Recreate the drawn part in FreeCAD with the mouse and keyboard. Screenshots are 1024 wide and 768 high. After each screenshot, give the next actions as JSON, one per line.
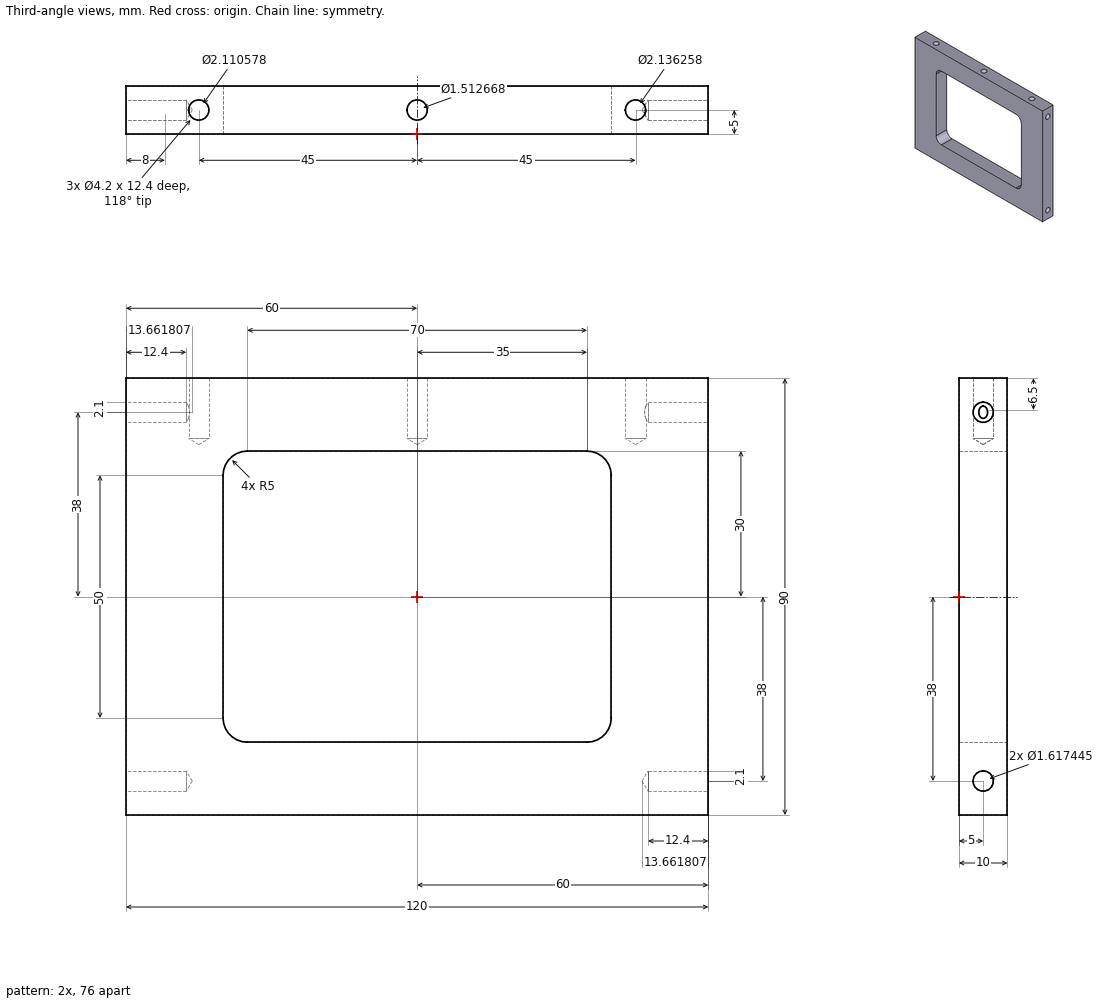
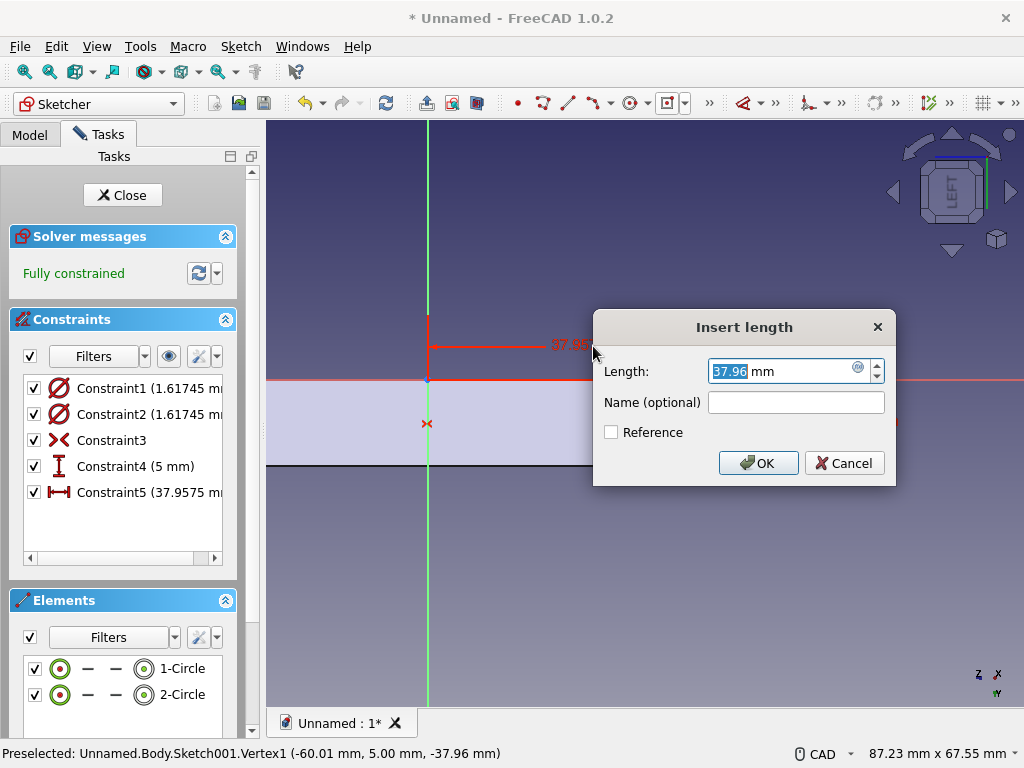
{"action": "type", "text": "38"}
{"action": "key", "text": "Return"}
{"action": "key", "text": "Escape"}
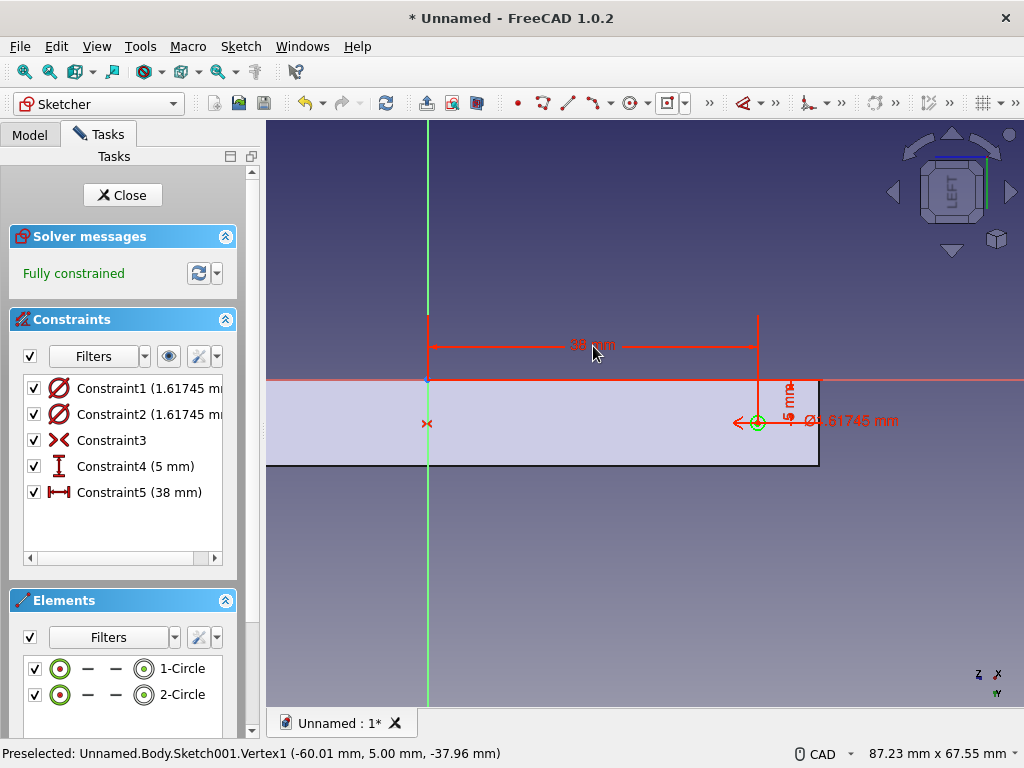
{"action": "left_click", "coordinate": [123, 195]}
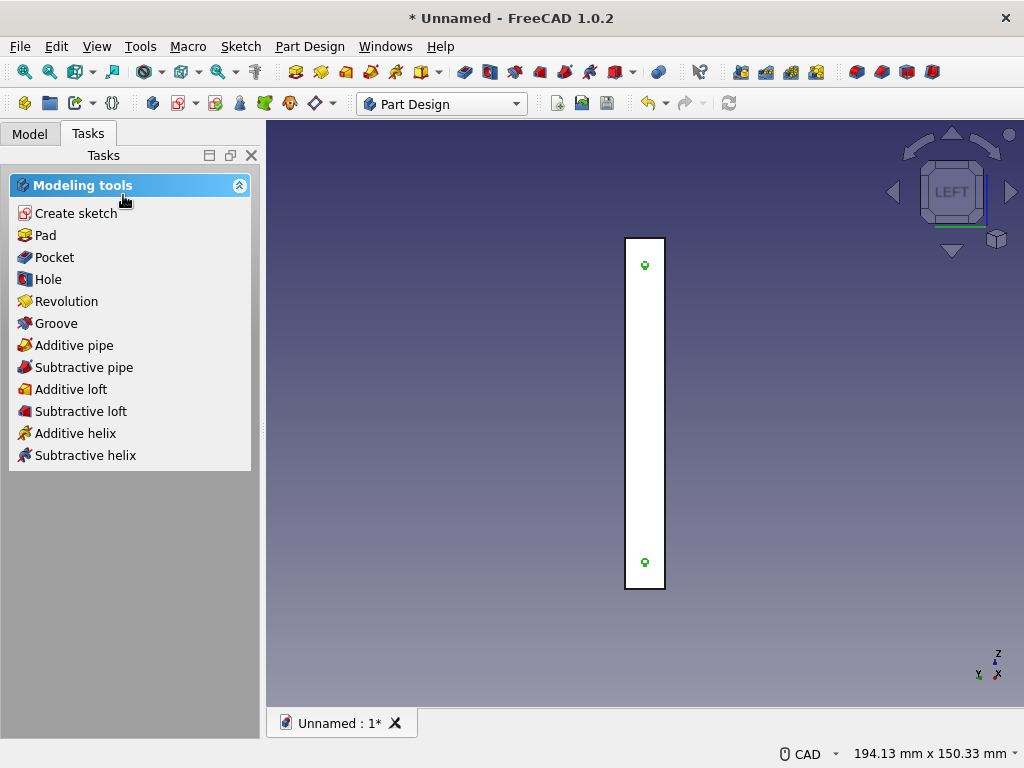
{"action": "left_click", "coordinate": [465, 72]}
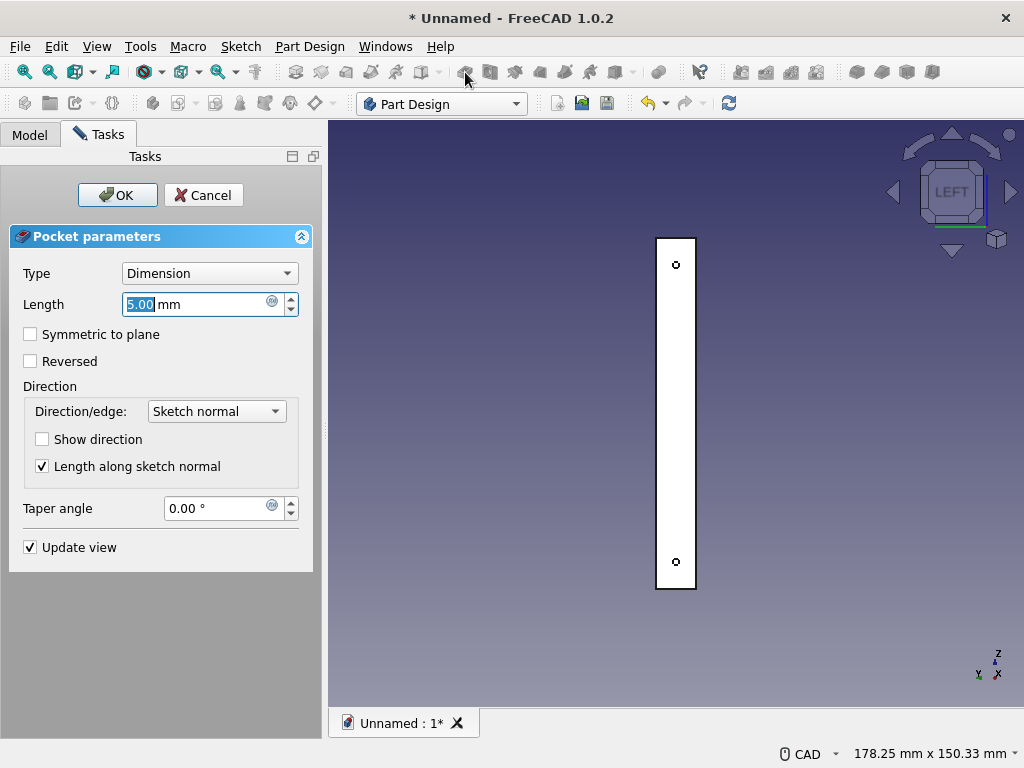
{"action": "type", "text": "8"}
{"action": "key", "text": "Tab"}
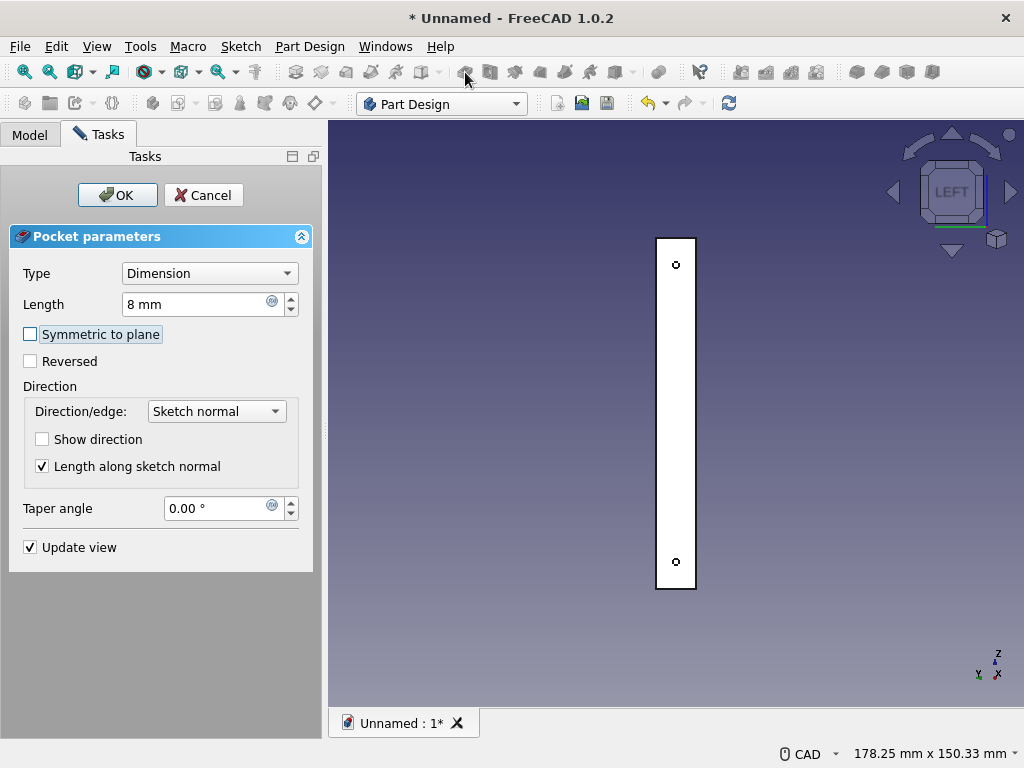
{"action": "left_click", "coordinate": [118, 195]}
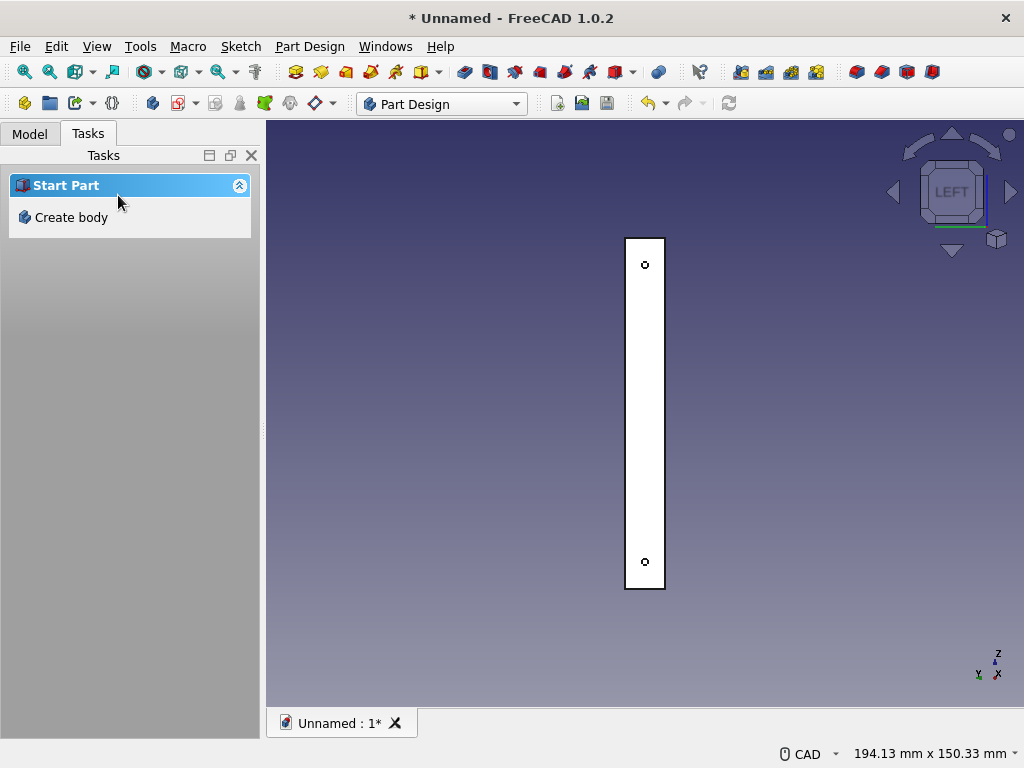
{"action": "left_click", "coordinate": [30, 134]}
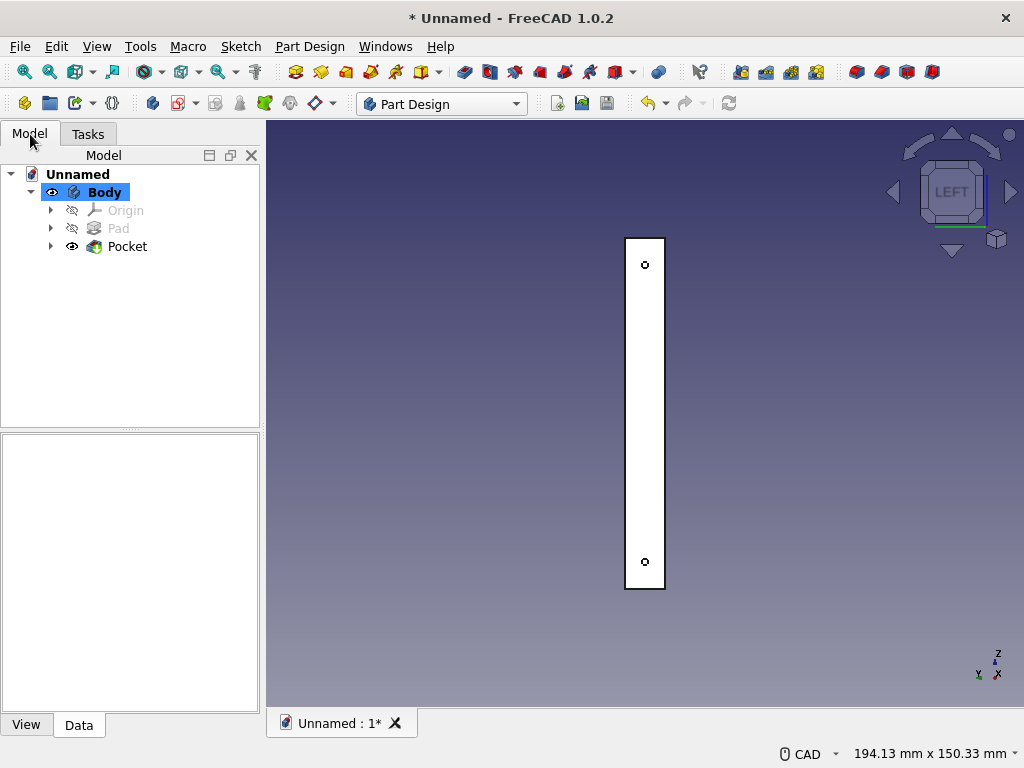
{"action": "left_click", "coordinate": [51, 210]}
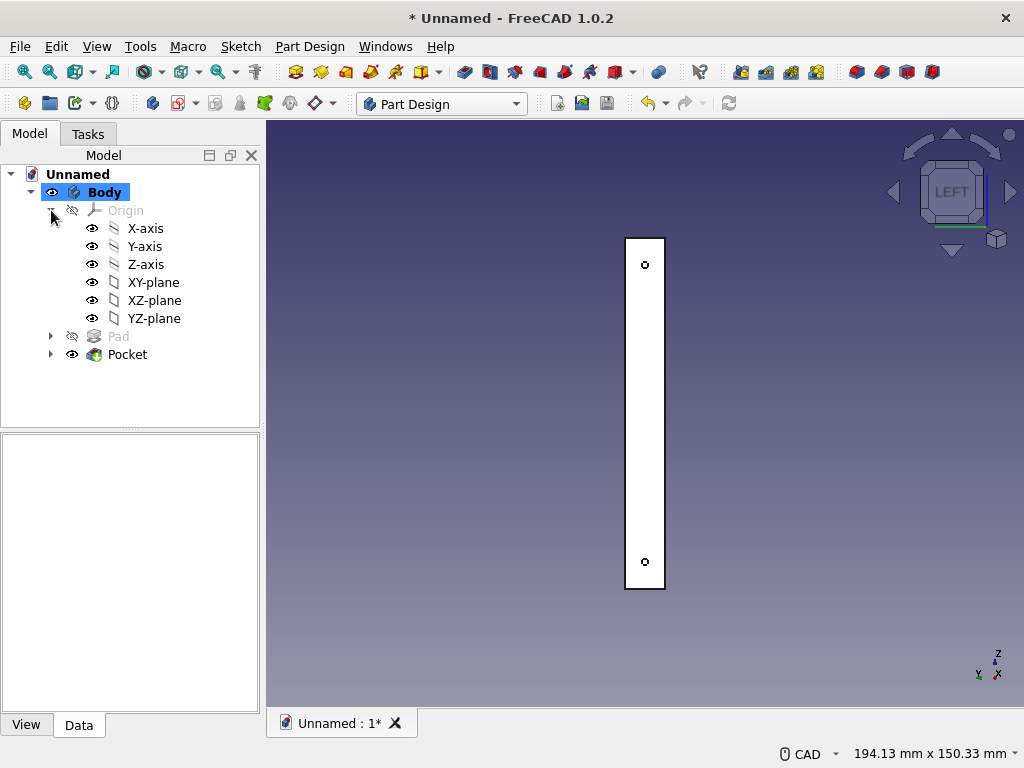
{"action": "left_click", "coordinate": [137, 300]}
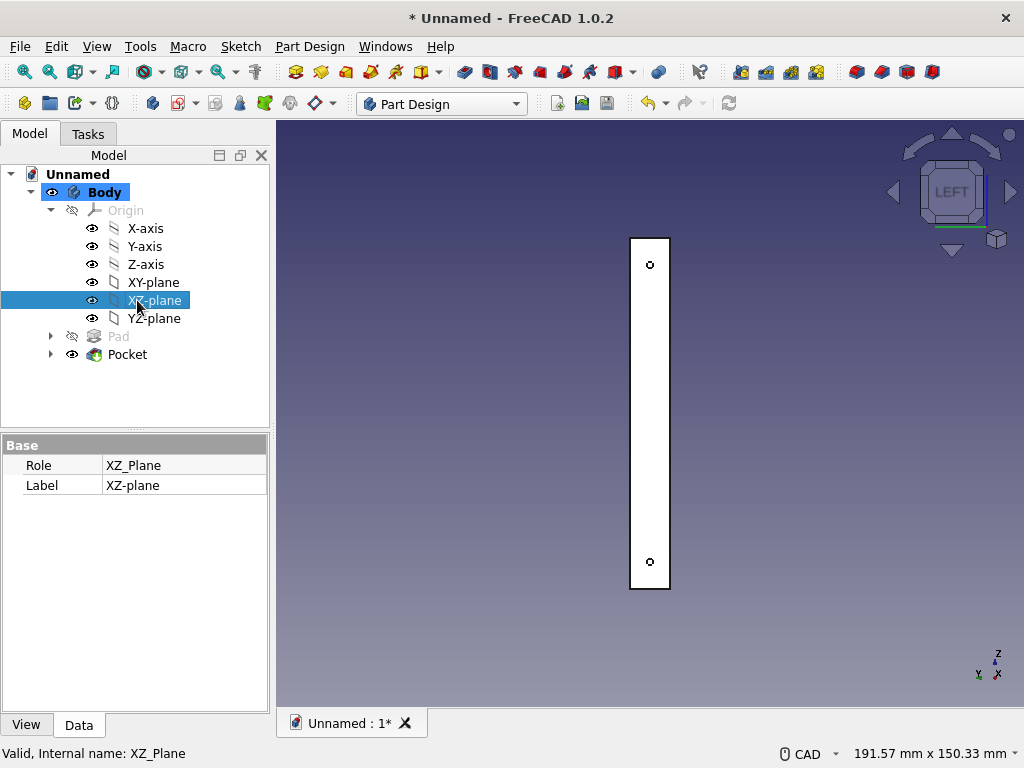
{"action": "left_click", "coordinate": [314, 104]}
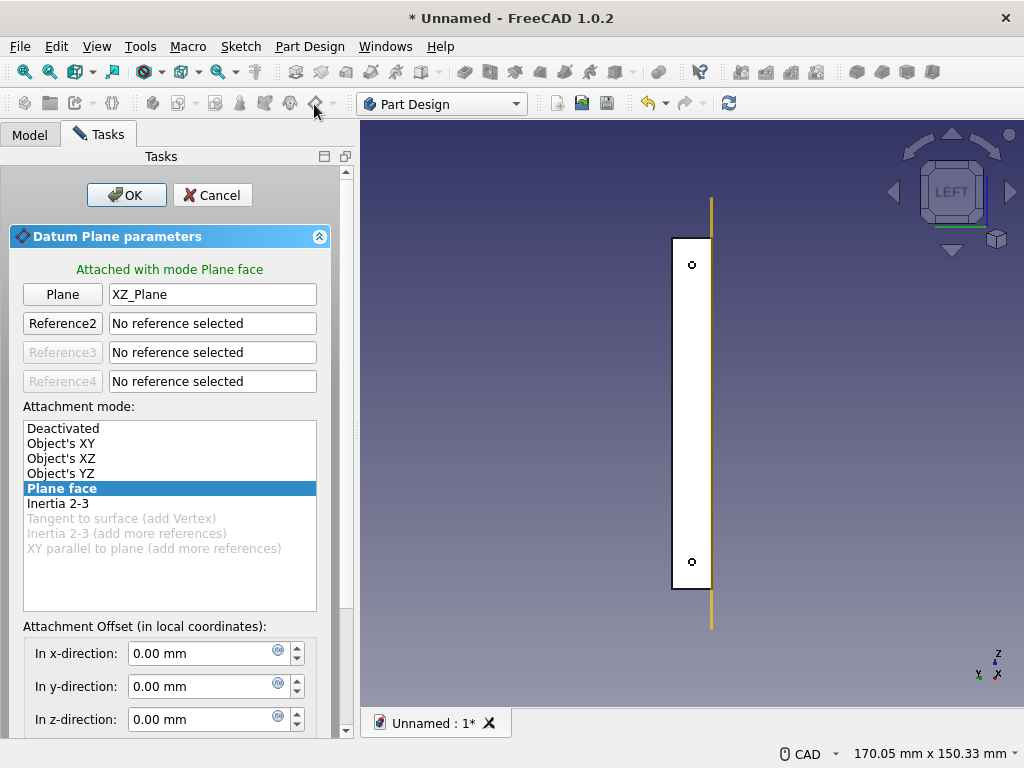
{"action": "triple_click", "coordinate": [210, 720]}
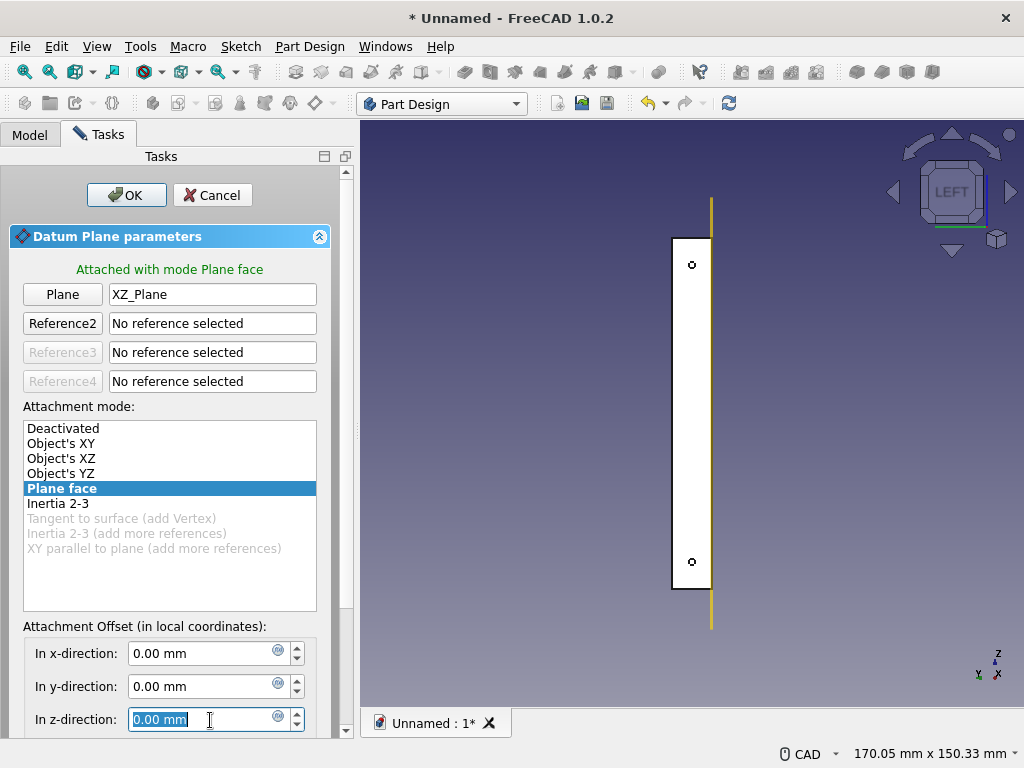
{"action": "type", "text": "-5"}
{"action": "key", "text": "Tab"}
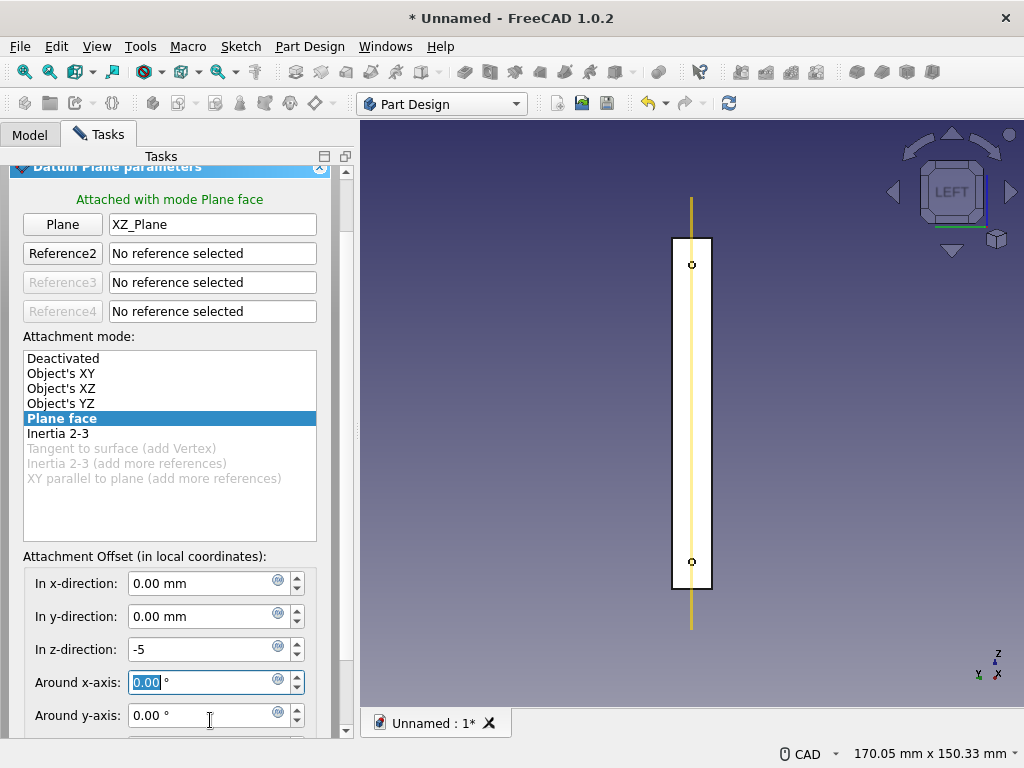
{"action": "scroll", "coordinate": [346, 452], "scroll_direction": "up", "scroll_amount": 2}